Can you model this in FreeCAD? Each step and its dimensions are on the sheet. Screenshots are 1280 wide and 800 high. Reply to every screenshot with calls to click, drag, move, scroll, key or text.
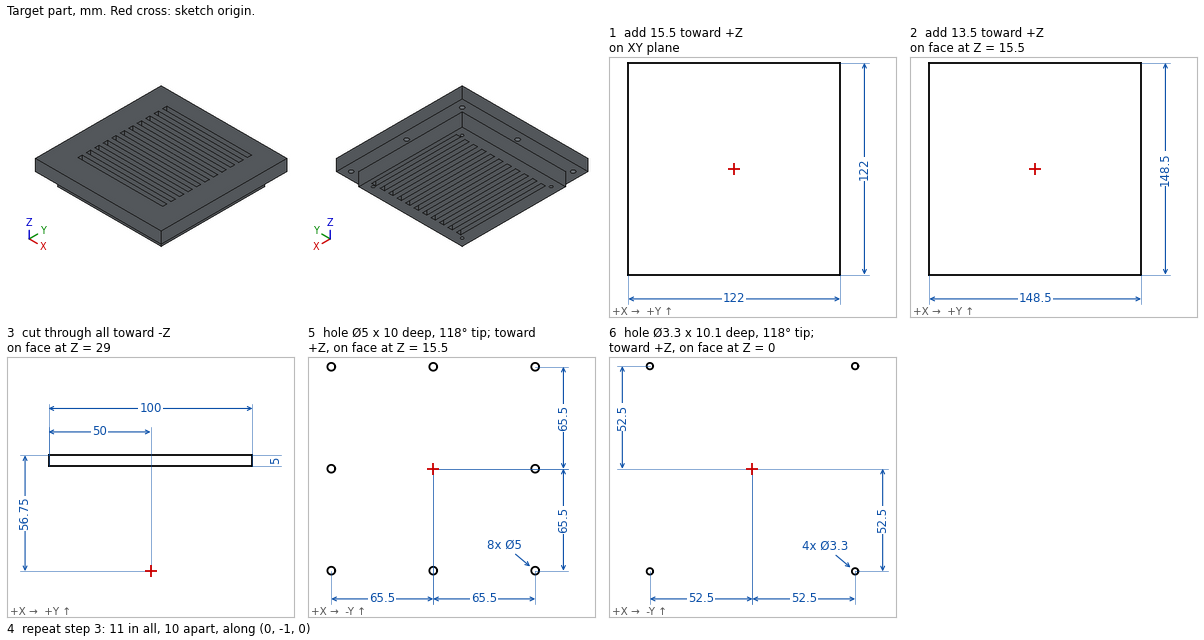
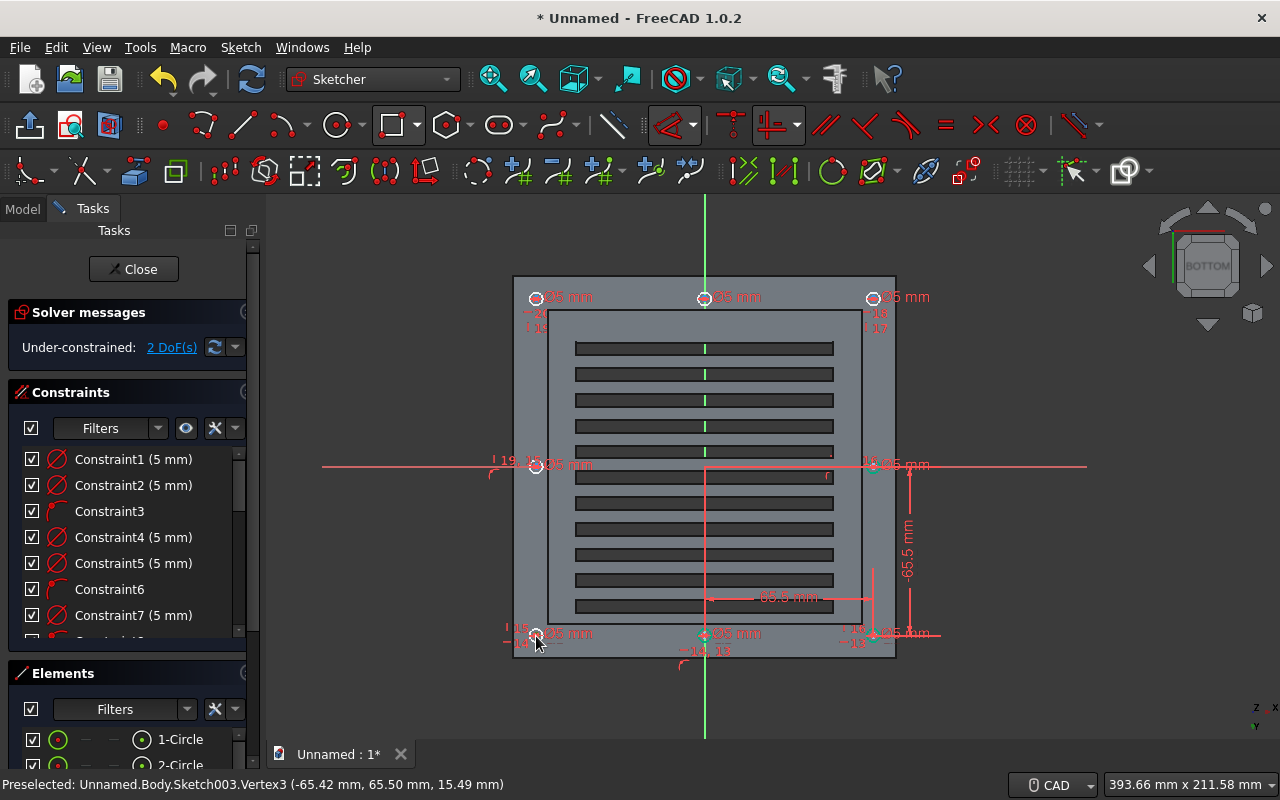
key(l)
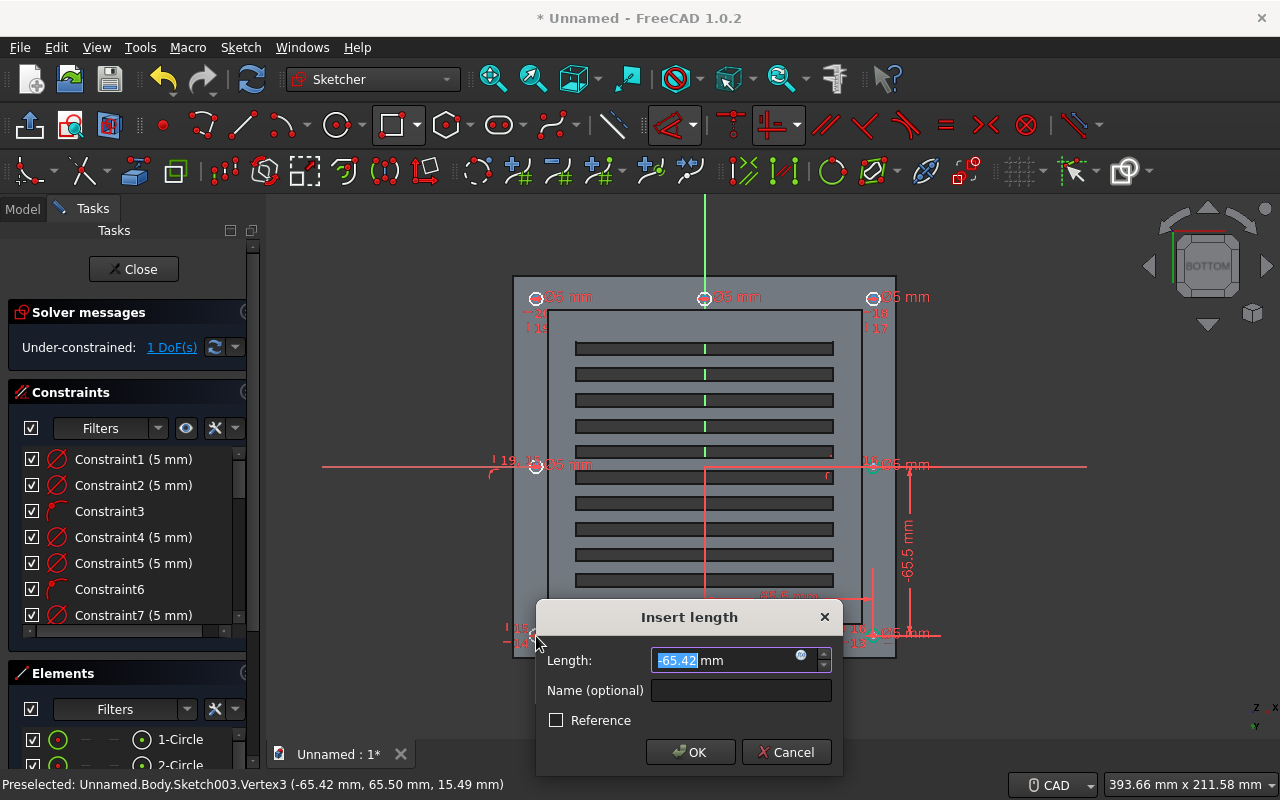
text(-65.5)
key(Return)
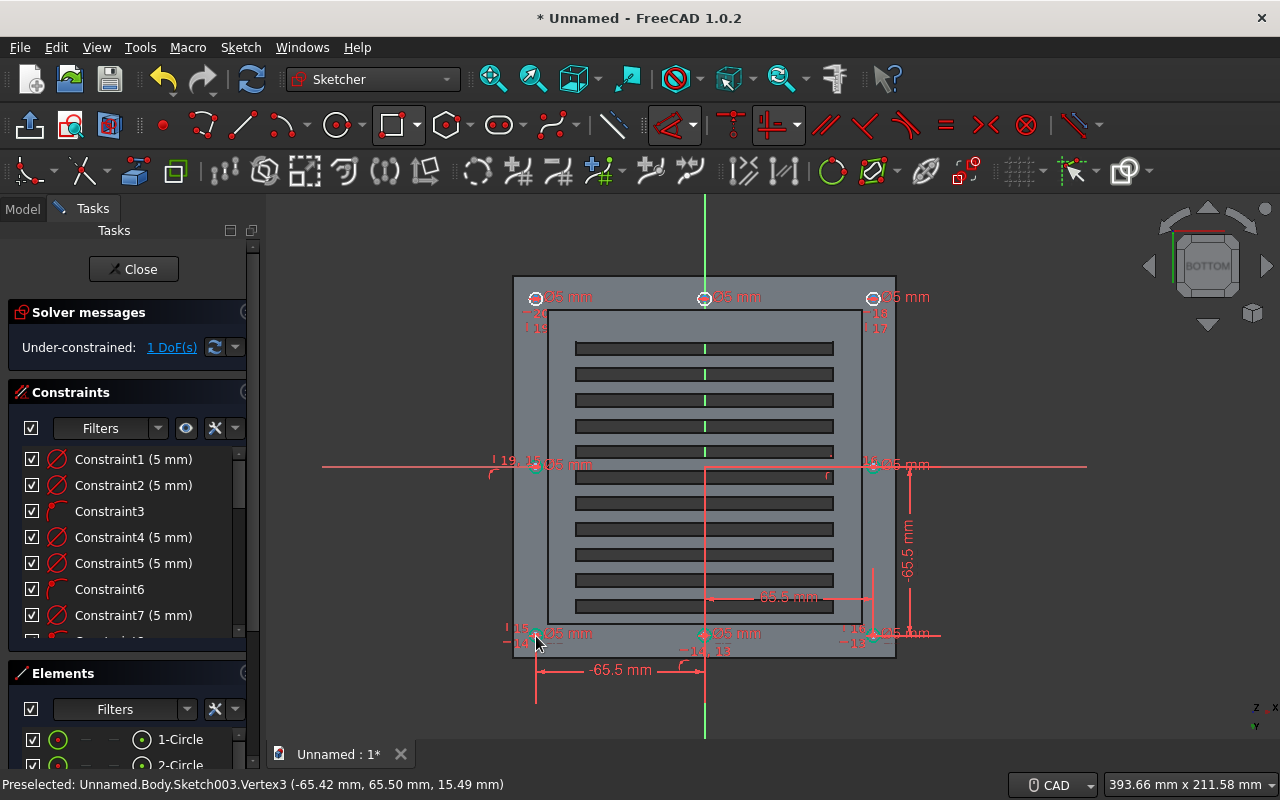
click(873, 299)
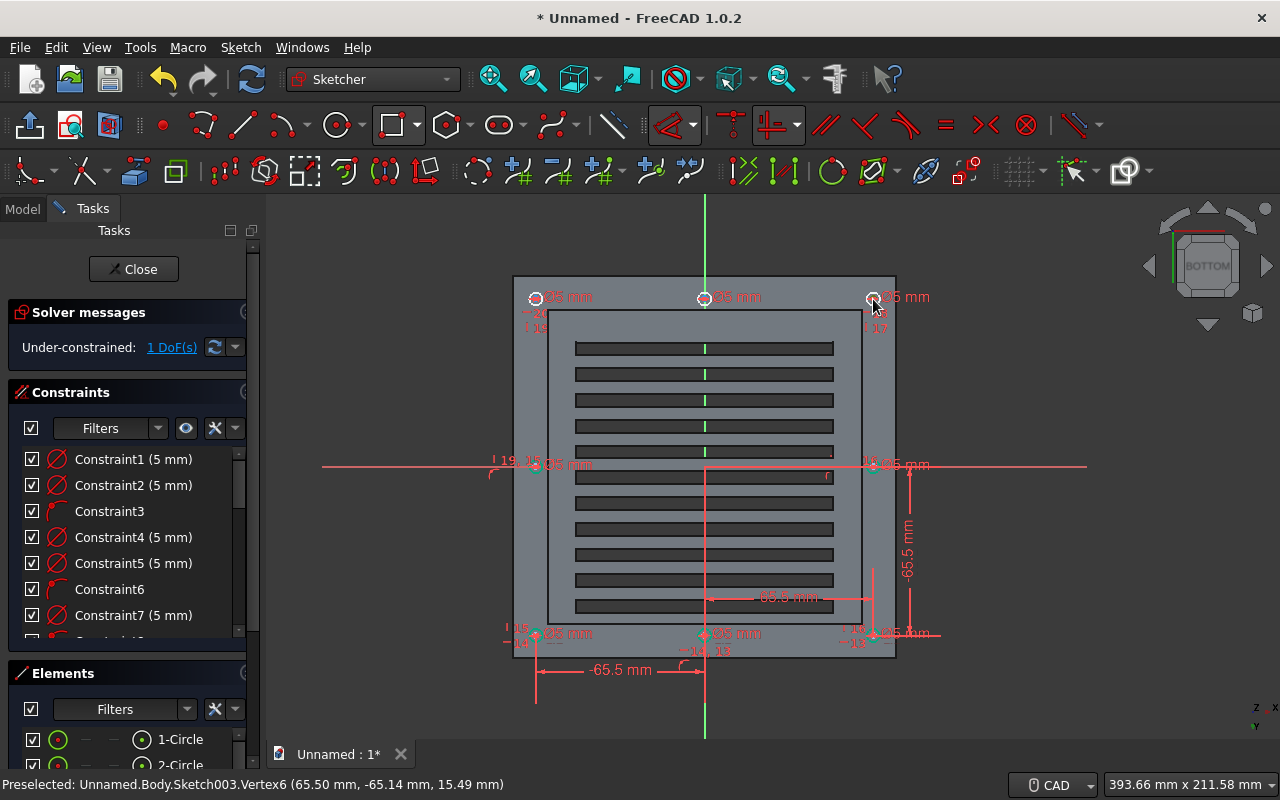
click(696, 126)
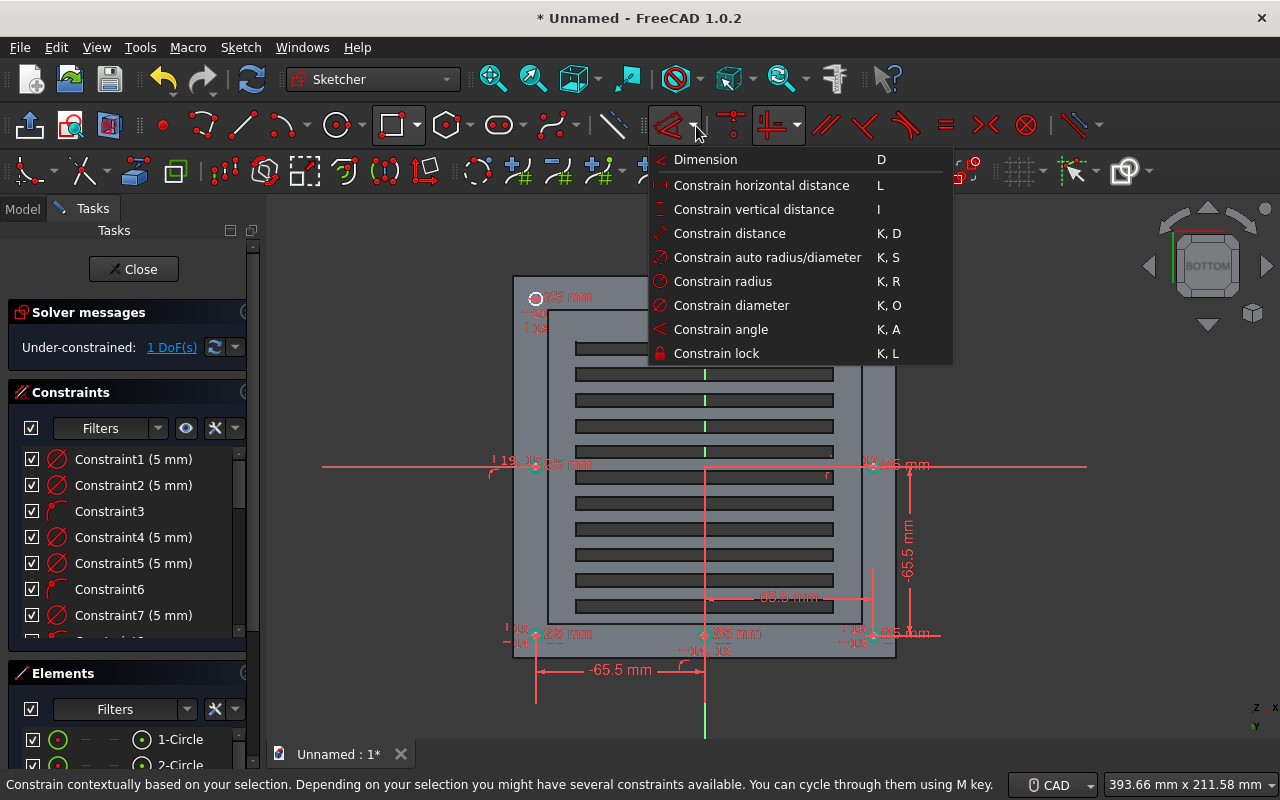
click(801, 209)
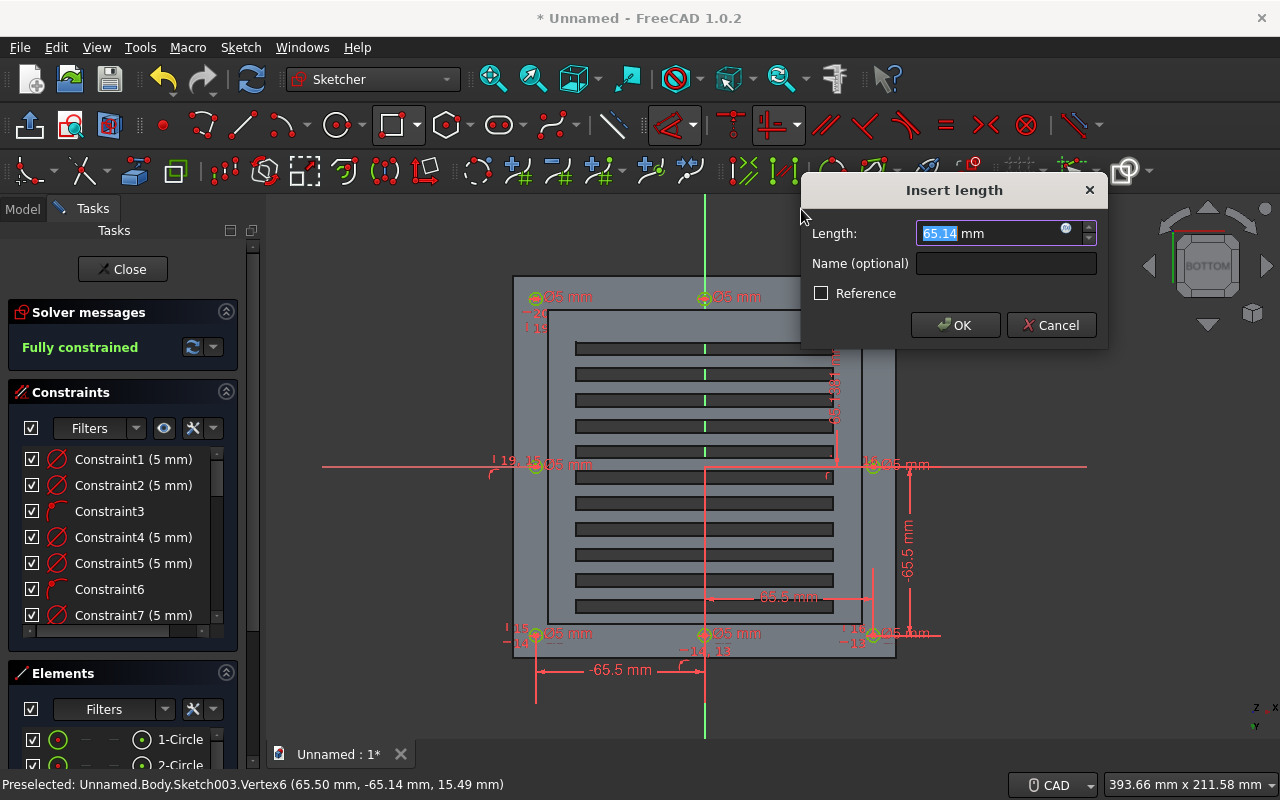
text(65.5)
key(Return)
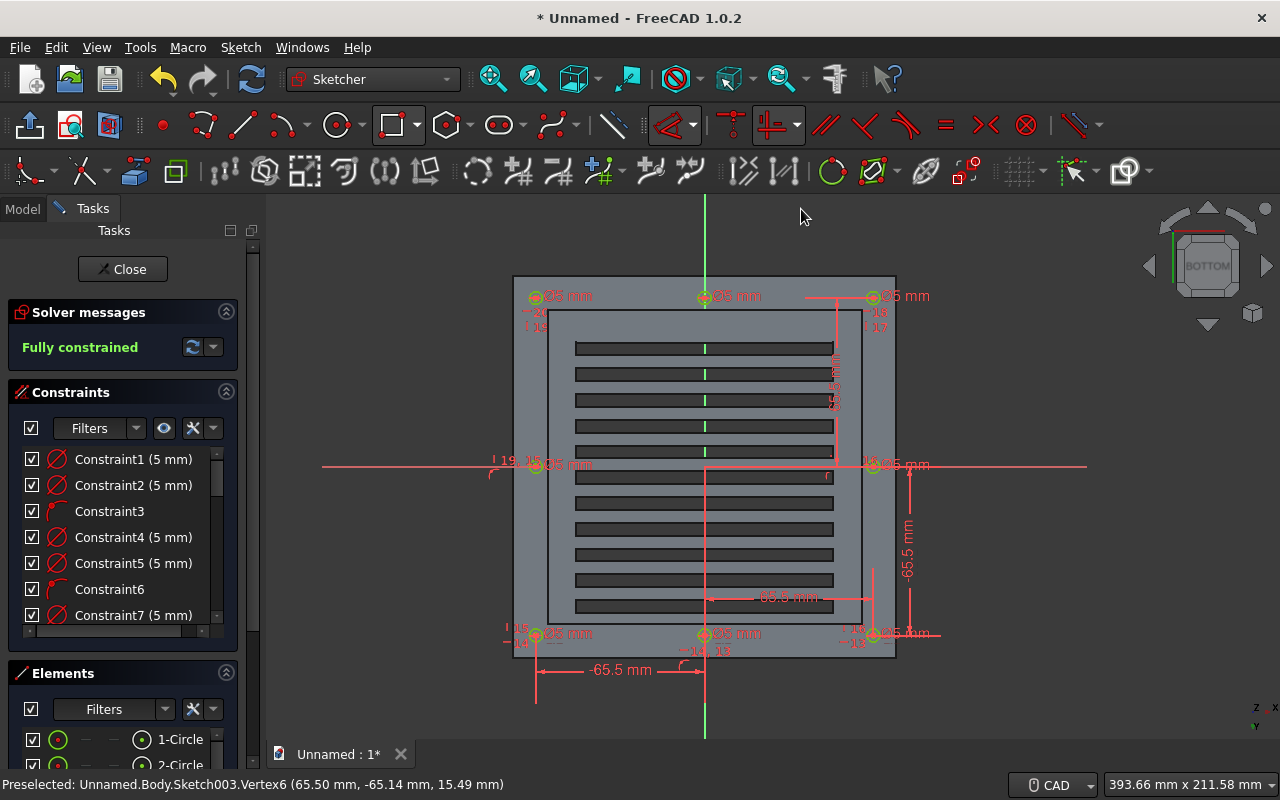
click(123, 269)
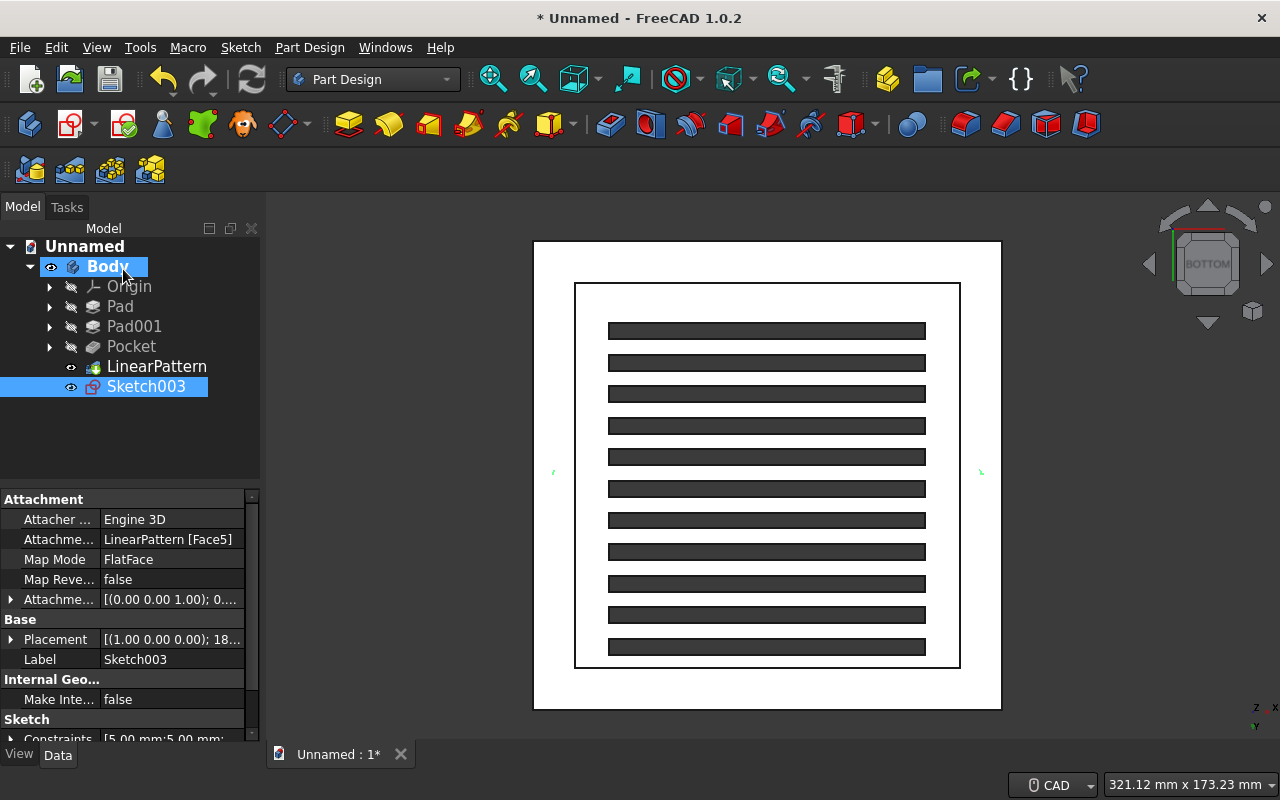
click(652, 124)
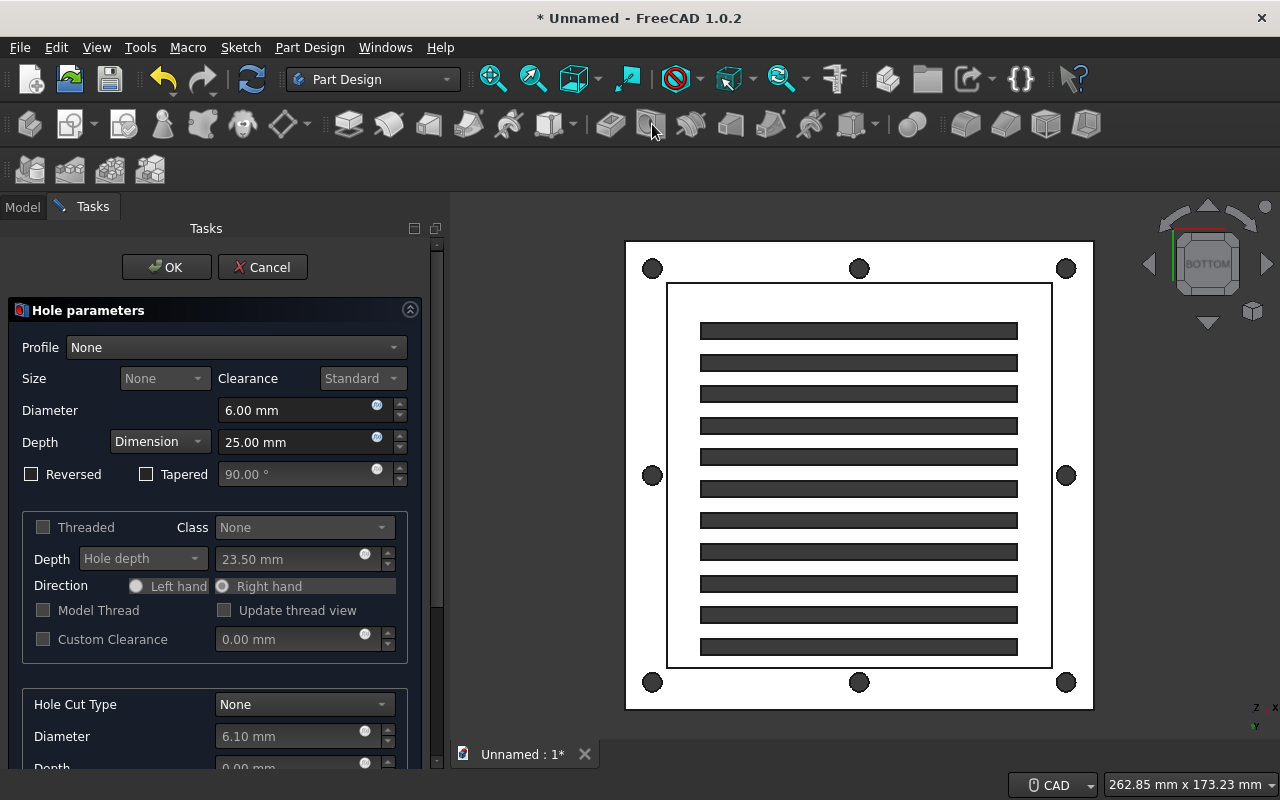
triple_click(305, 410)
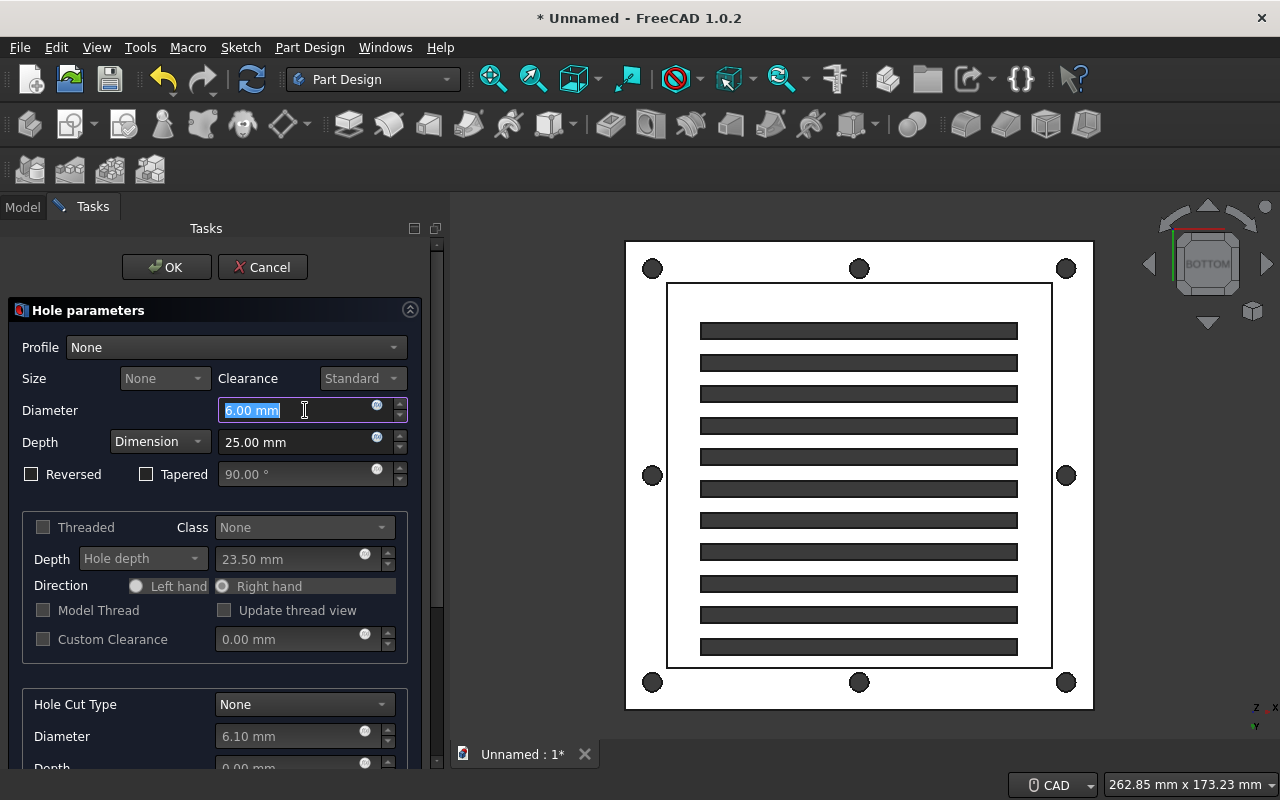
text(5)
key(Tab)